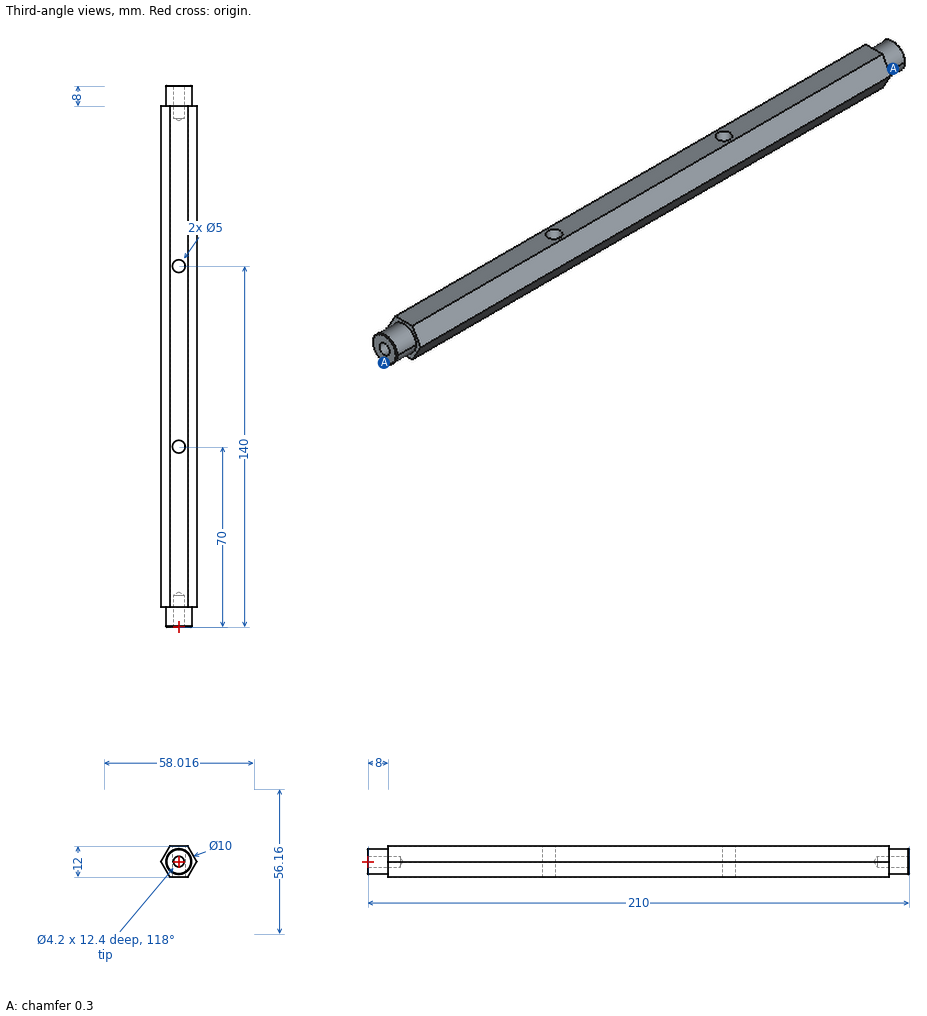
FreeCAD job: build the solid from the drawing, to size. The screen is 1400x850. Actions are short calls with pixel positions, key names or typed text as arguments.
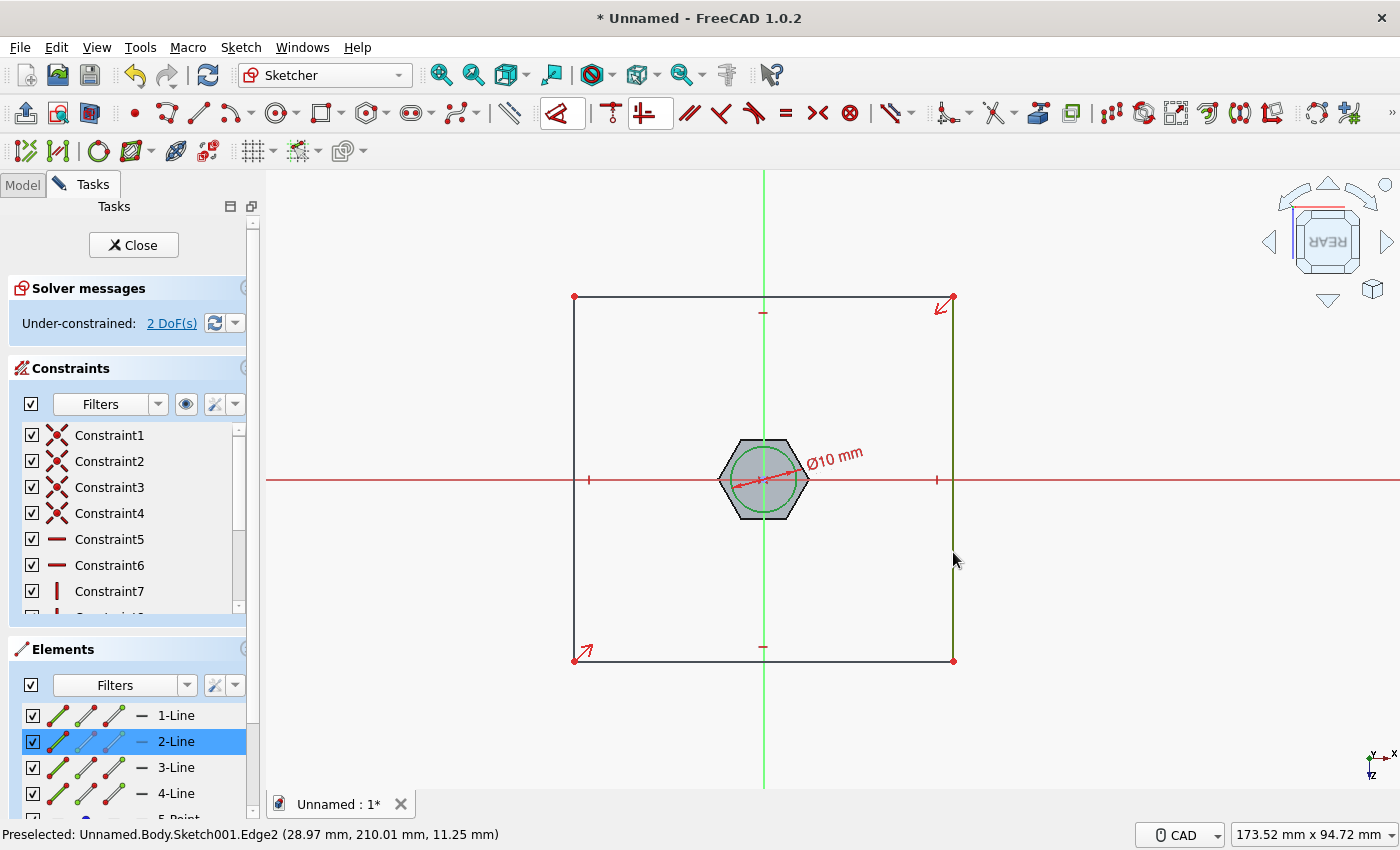
key(i)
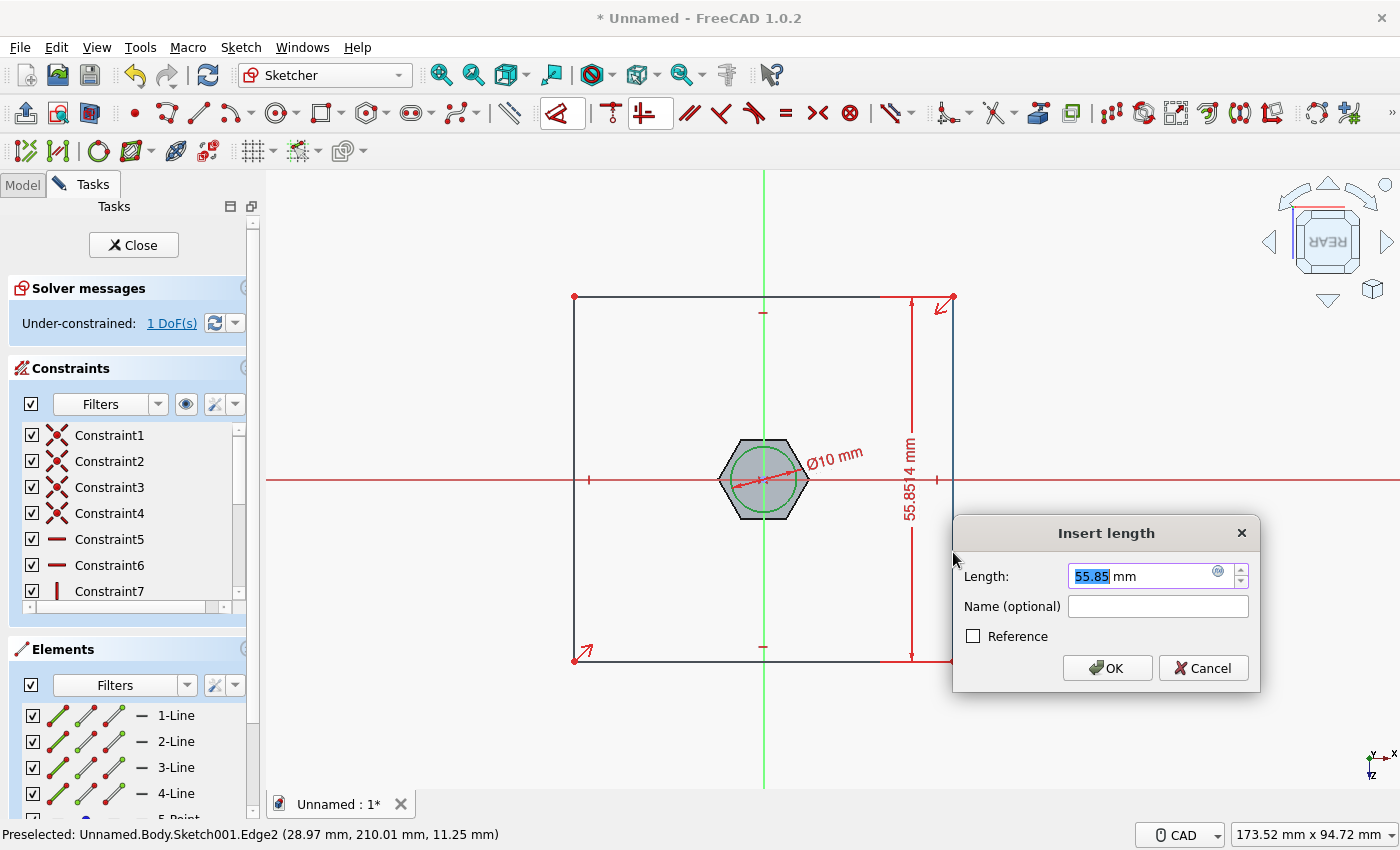
text(56.16)
key(Return)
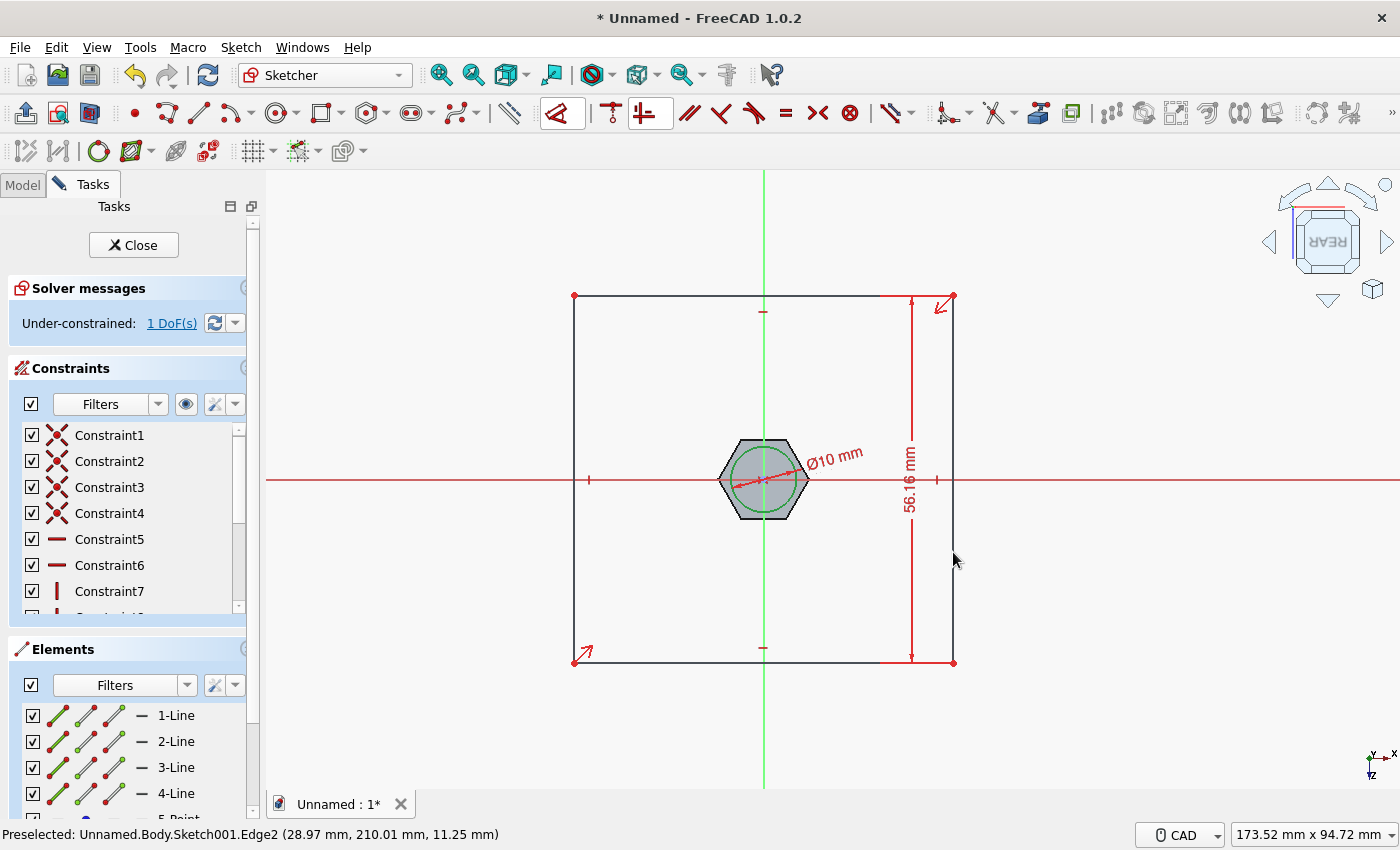
click(688, 663)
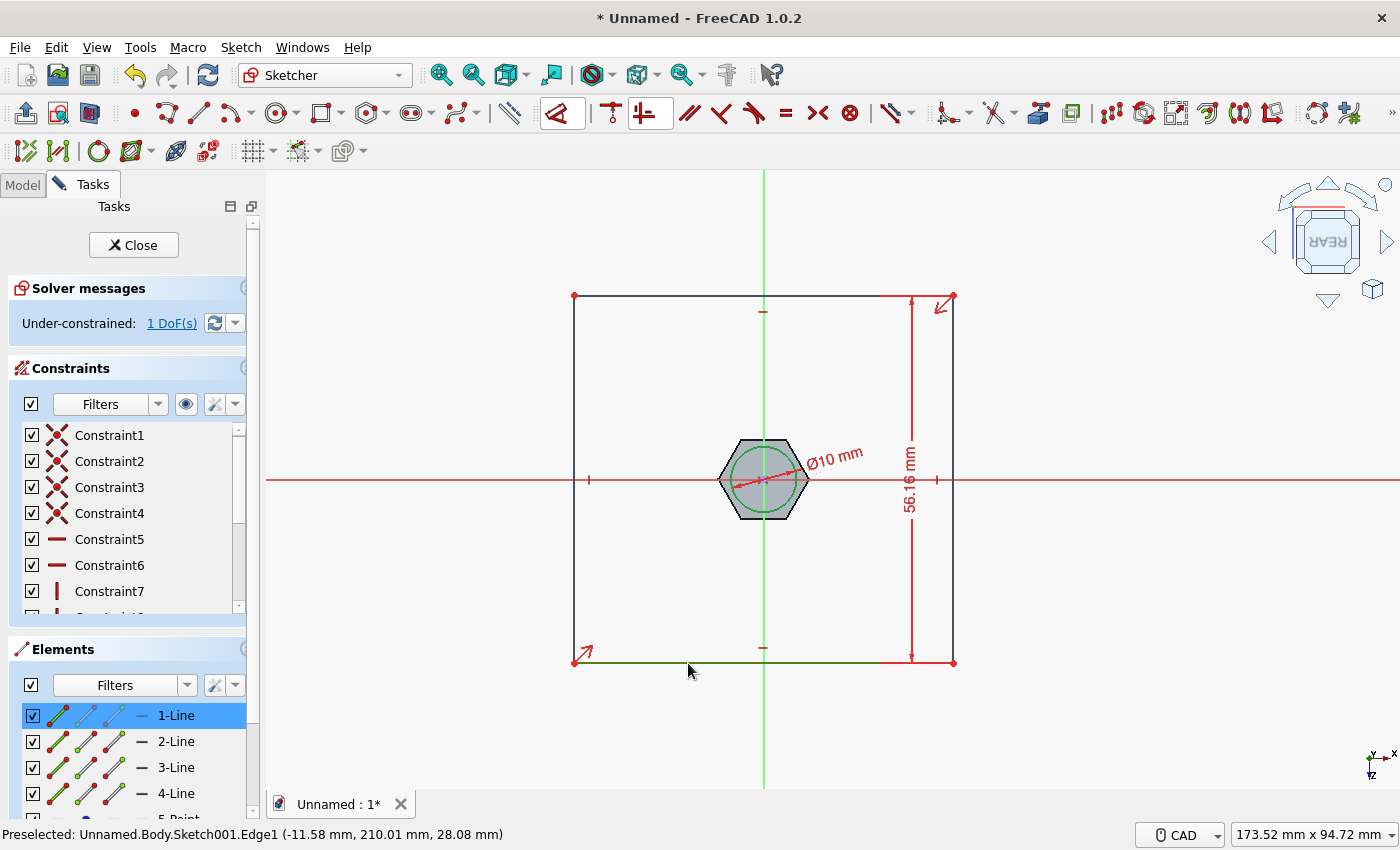
key(l)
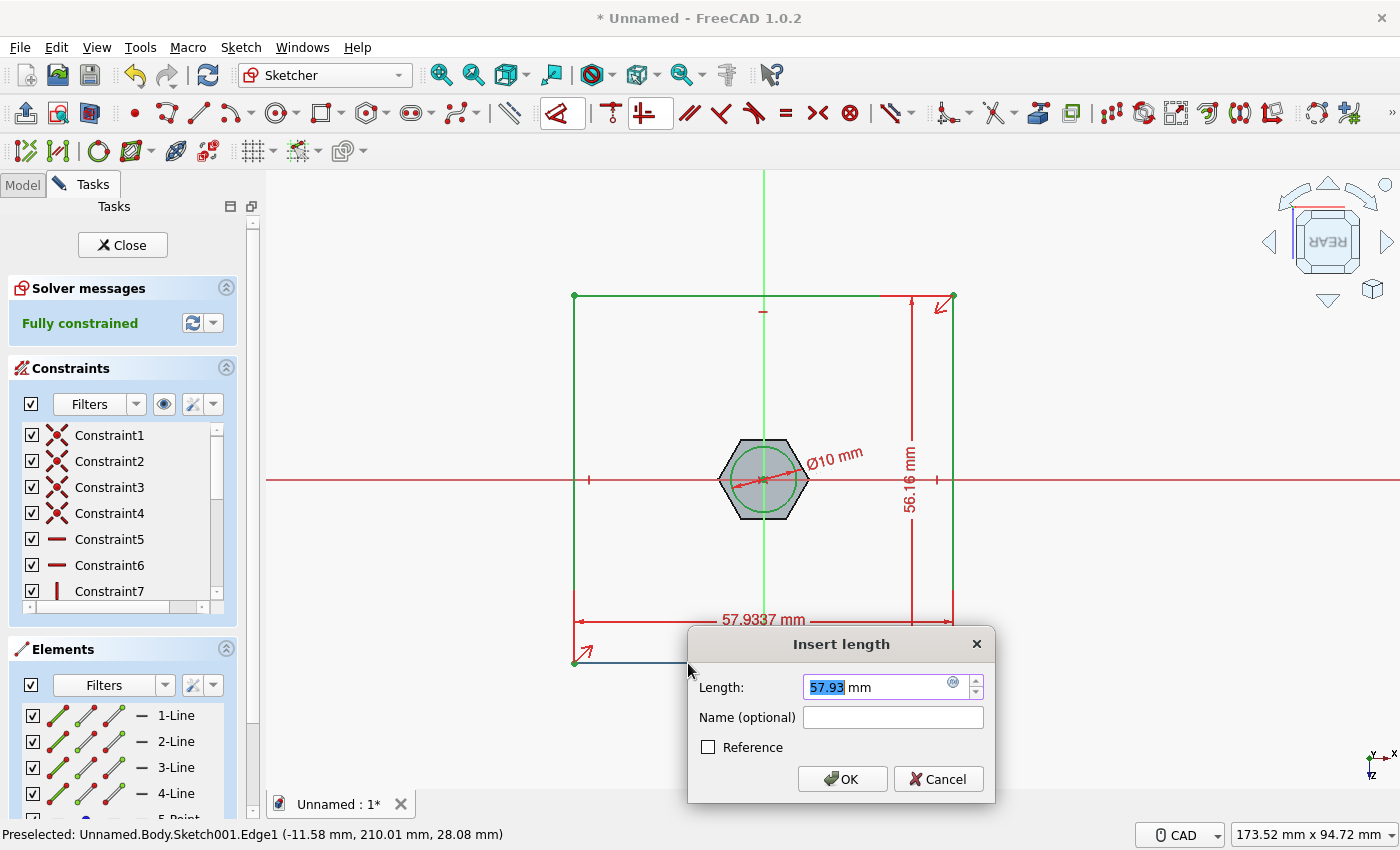
text(58.016)
key(Return)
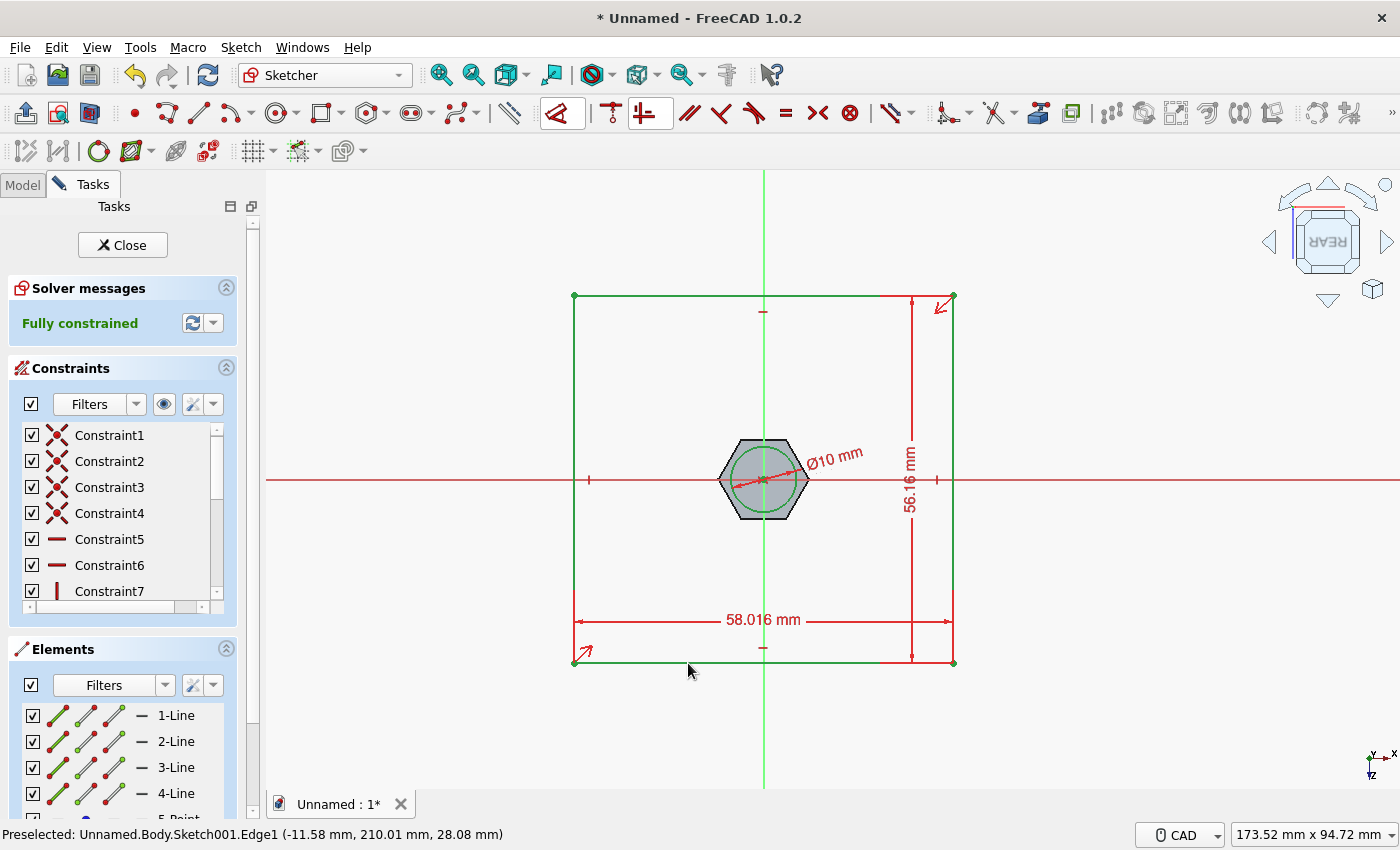
click(123, 245)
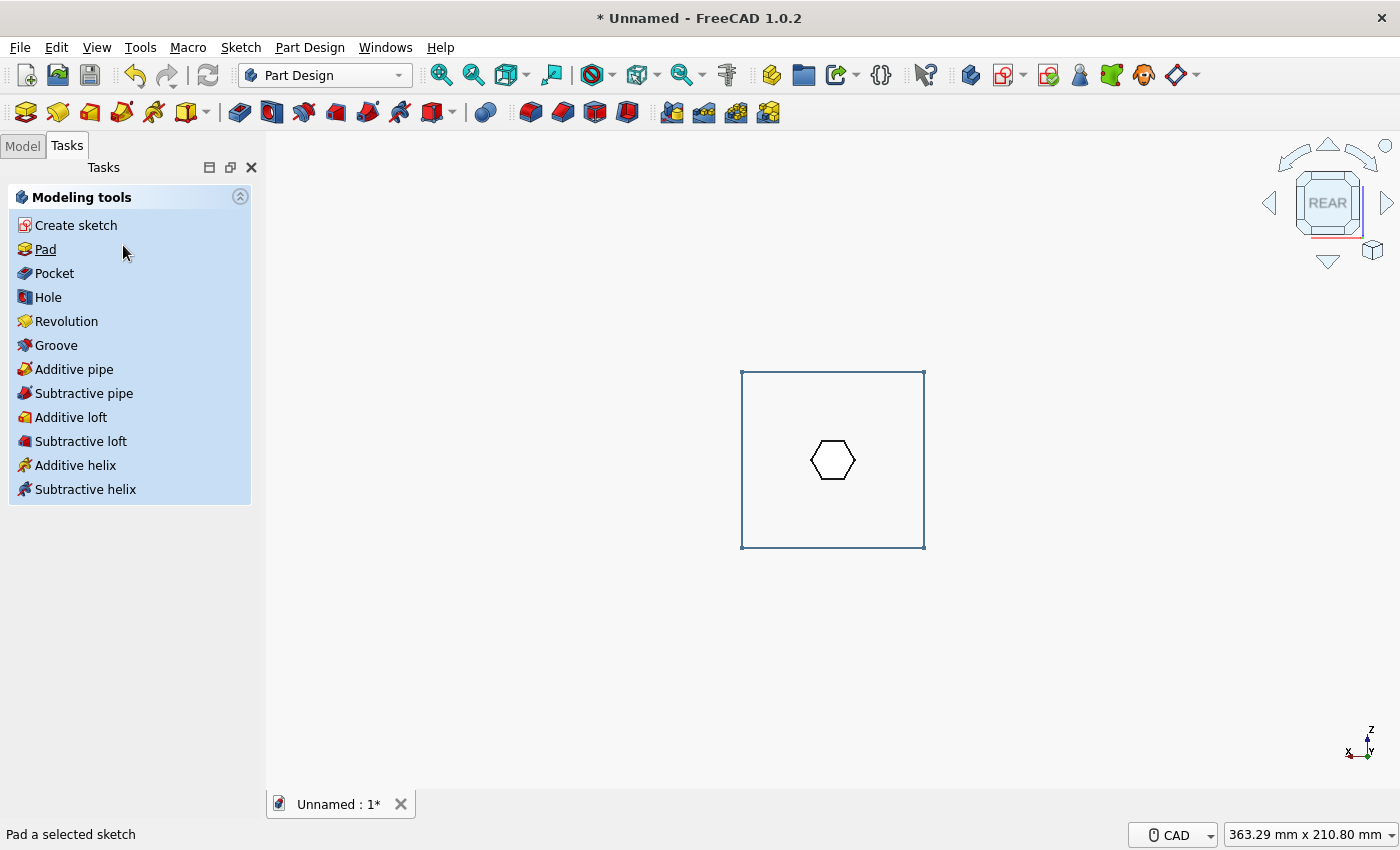
click(240, 112)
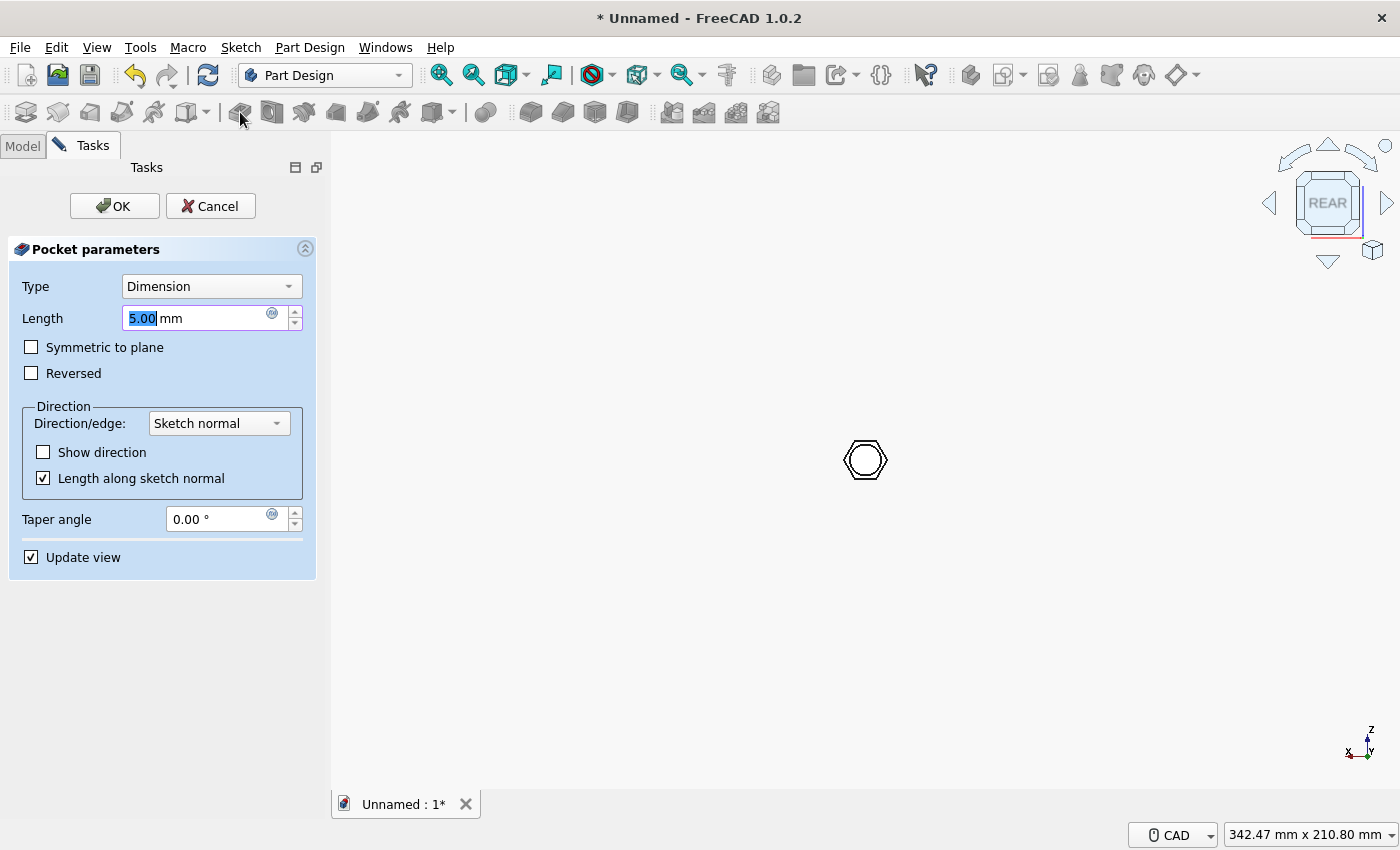
text(8)
key(Tab)